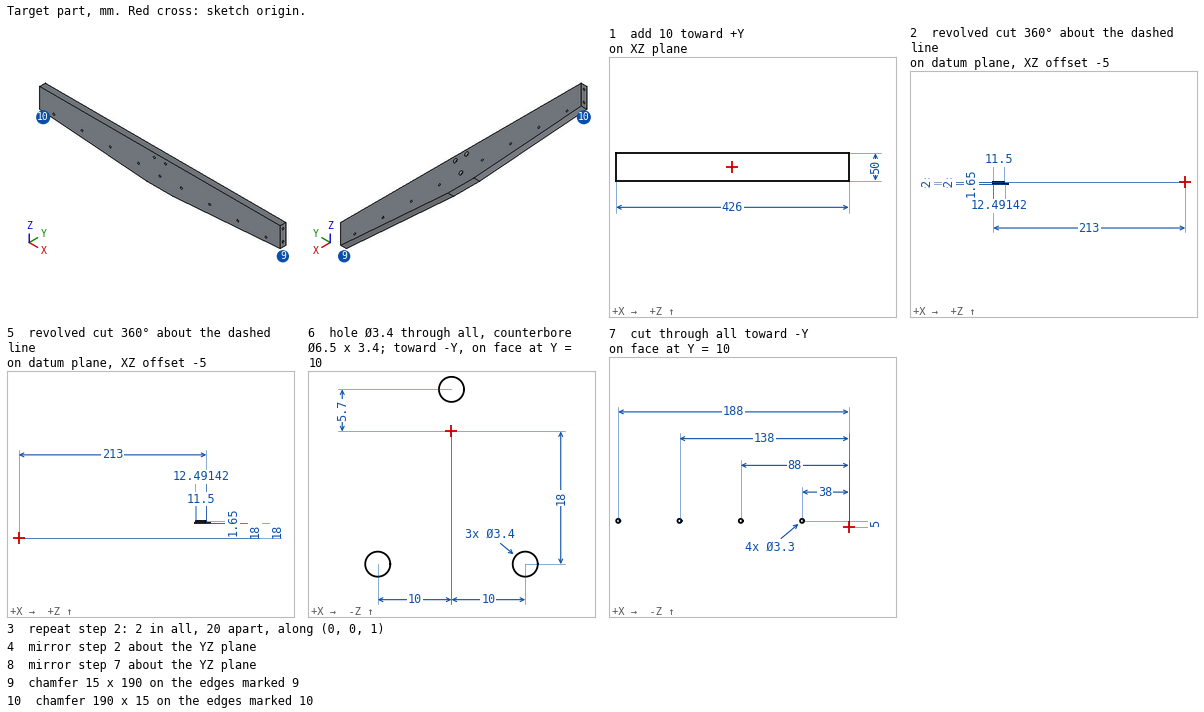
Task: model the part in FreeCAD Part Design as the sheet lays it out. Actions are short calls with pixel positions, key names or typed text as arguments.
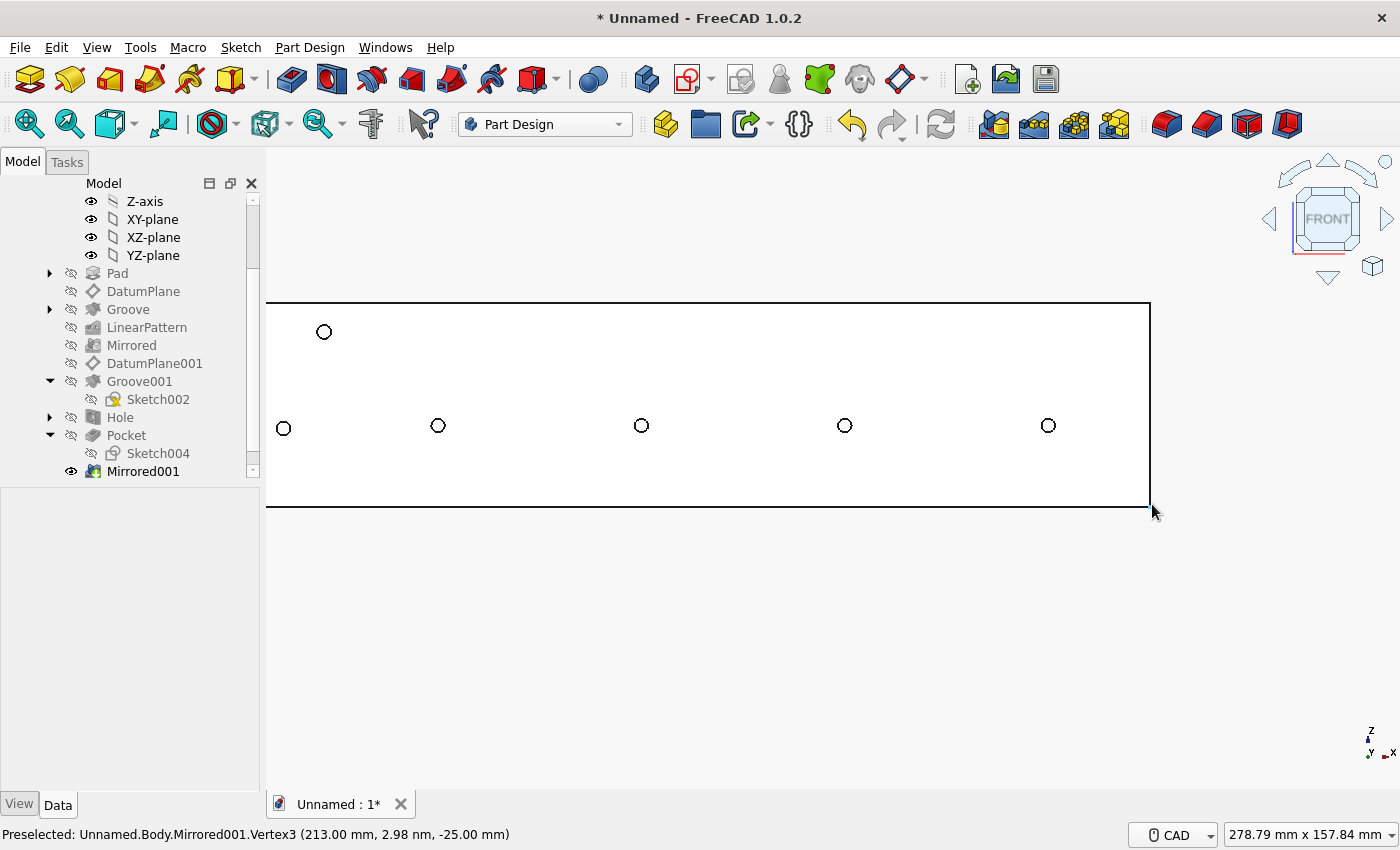
click(30, 124)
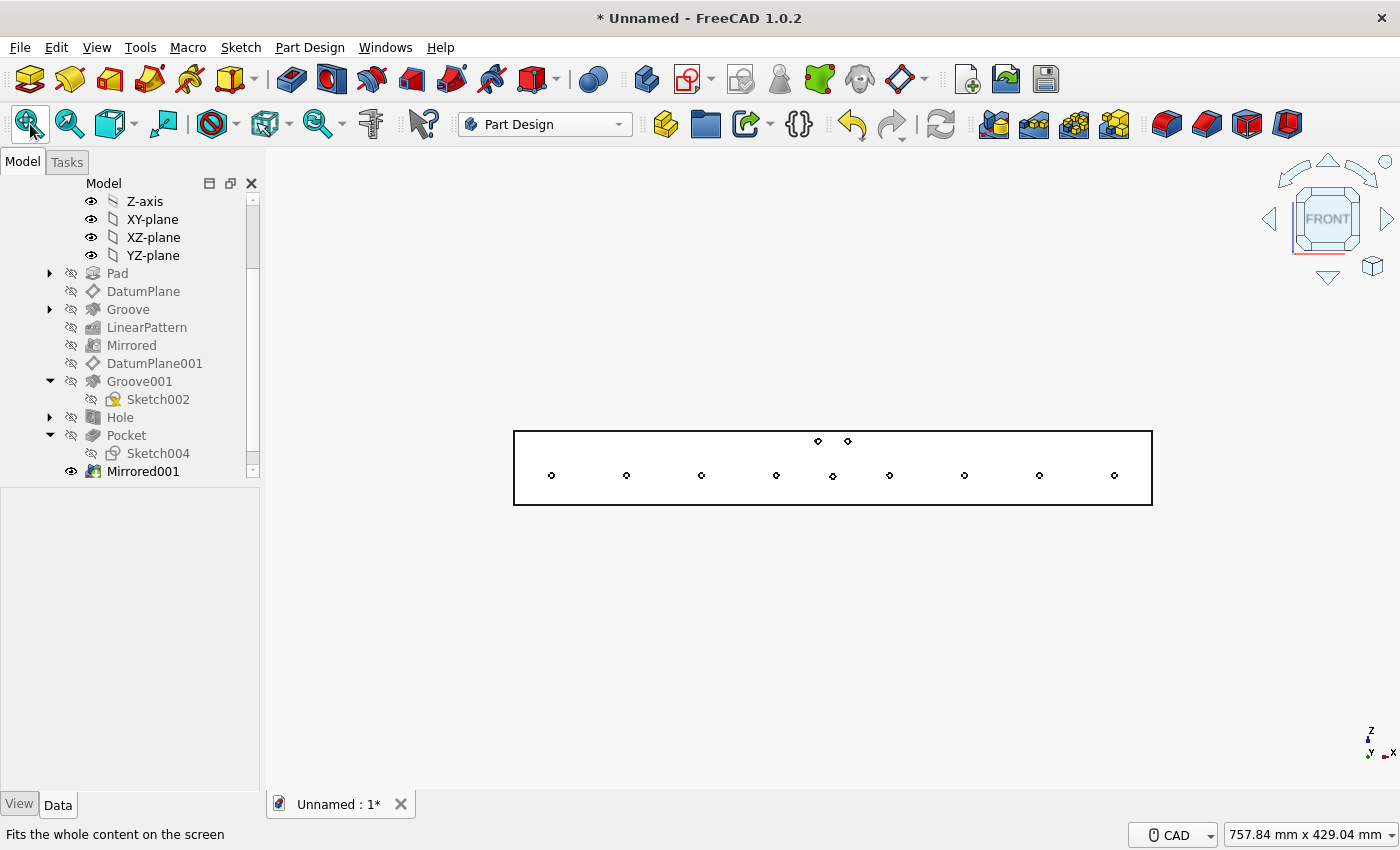
key(3)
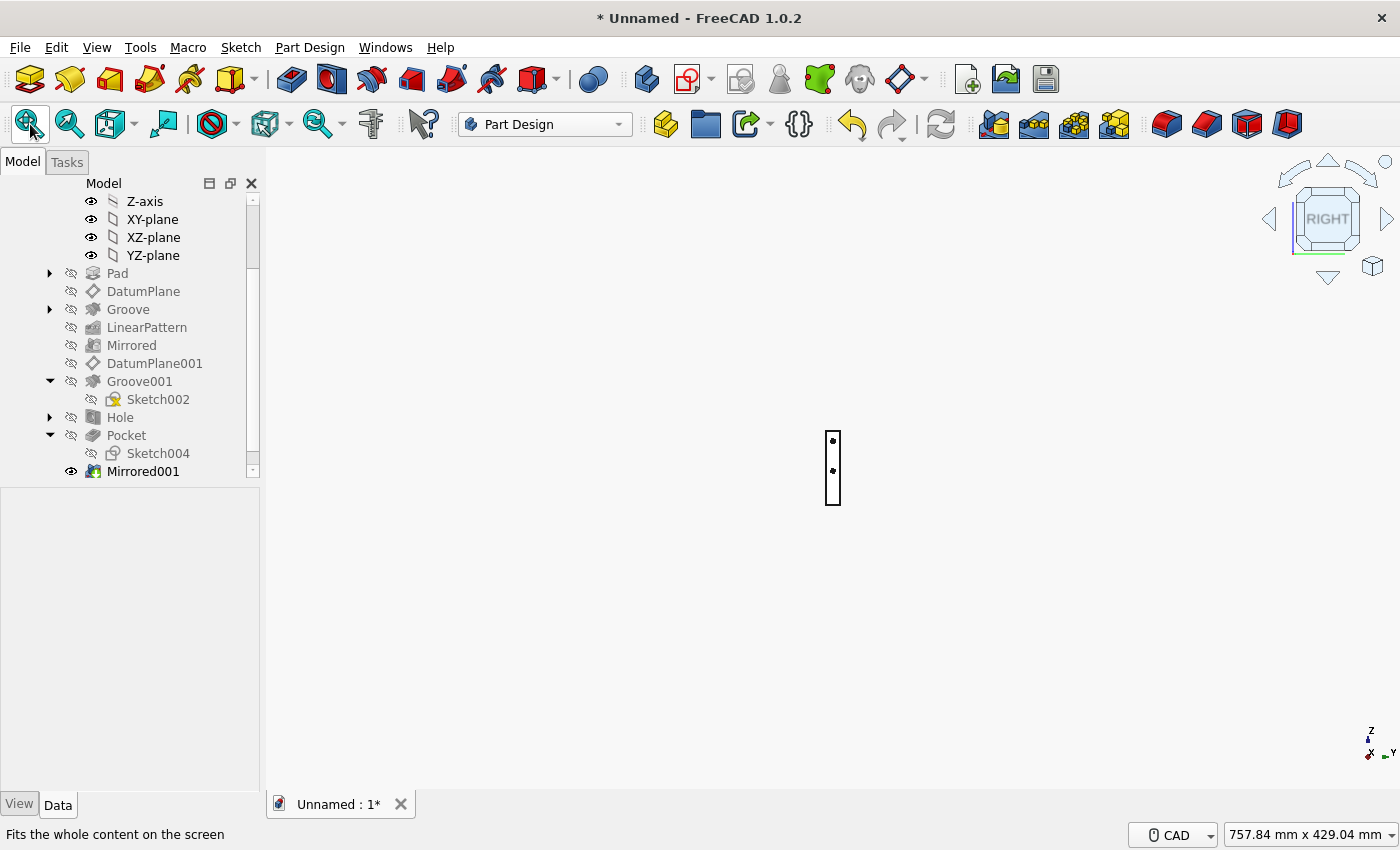
click(30, 124)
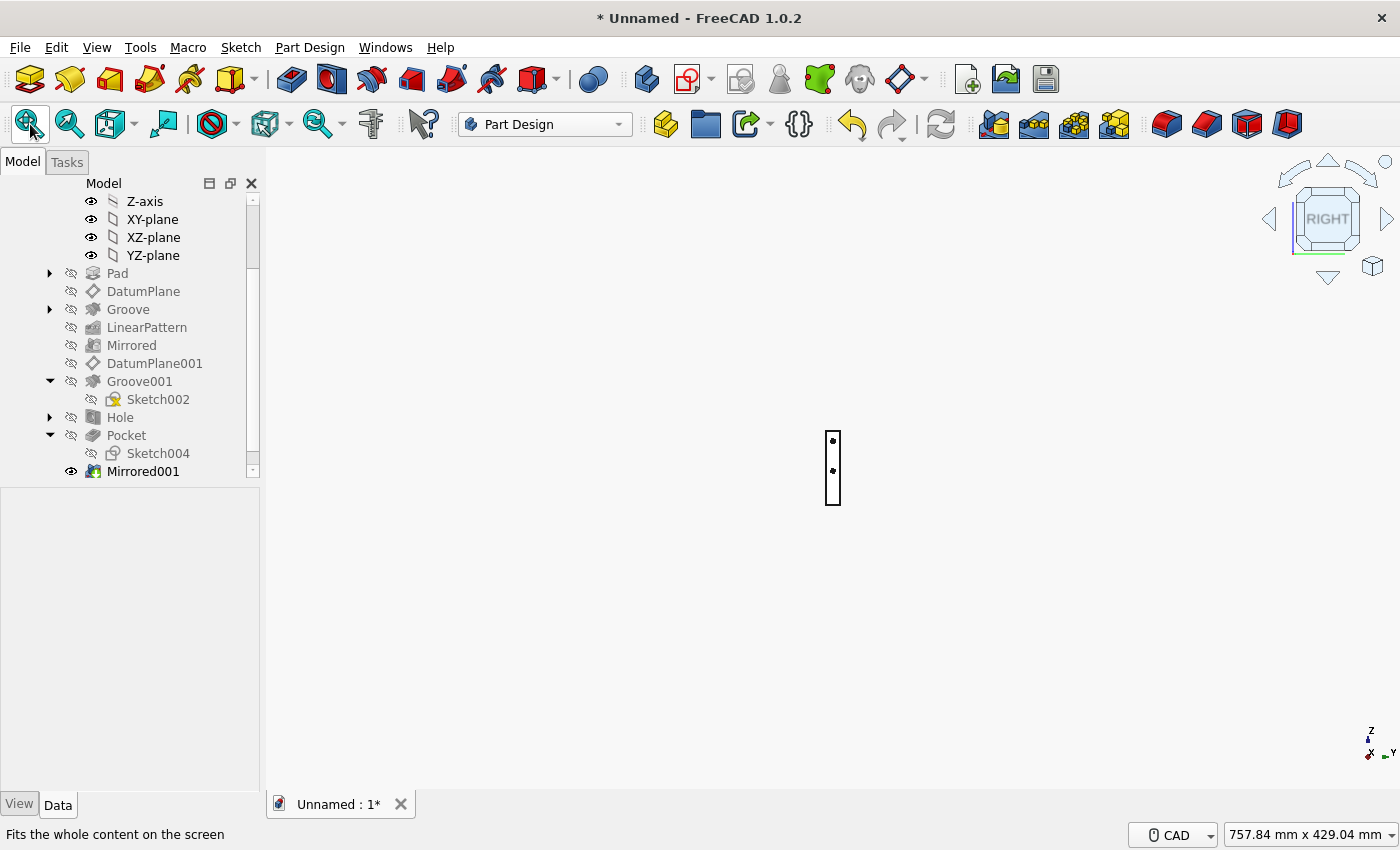
click(833, 504)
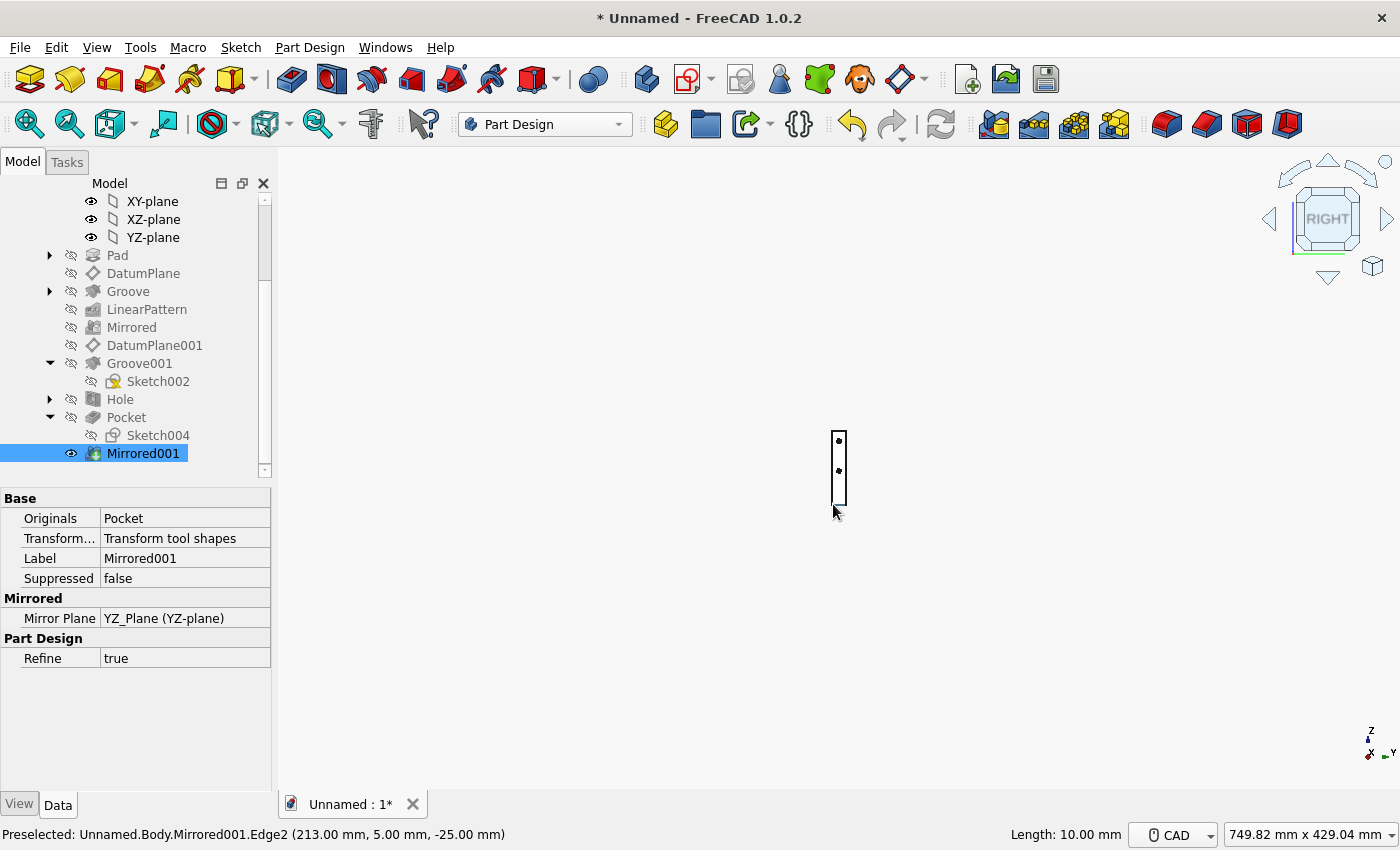
click(1208, 124)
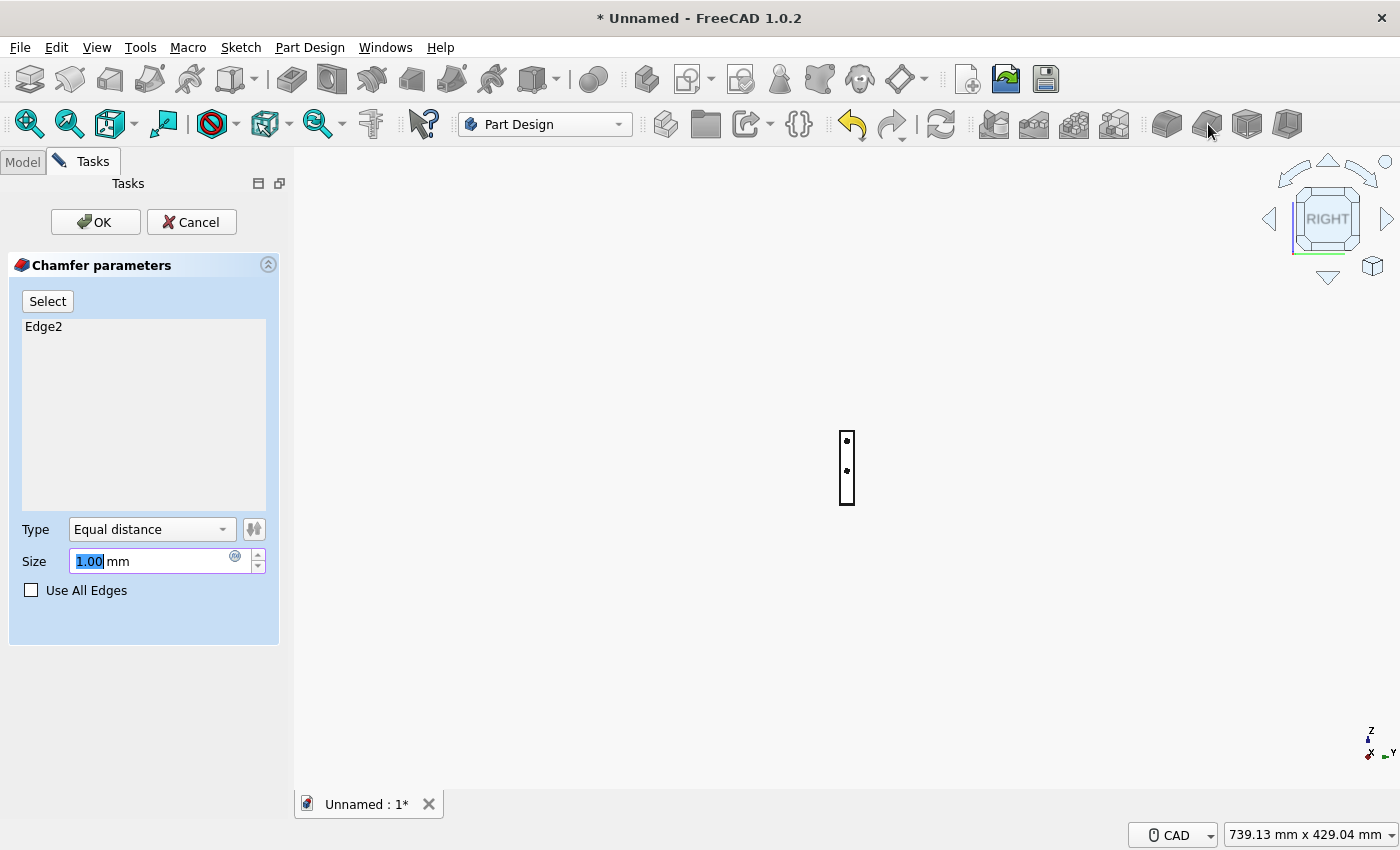
text(15)
key(Tab)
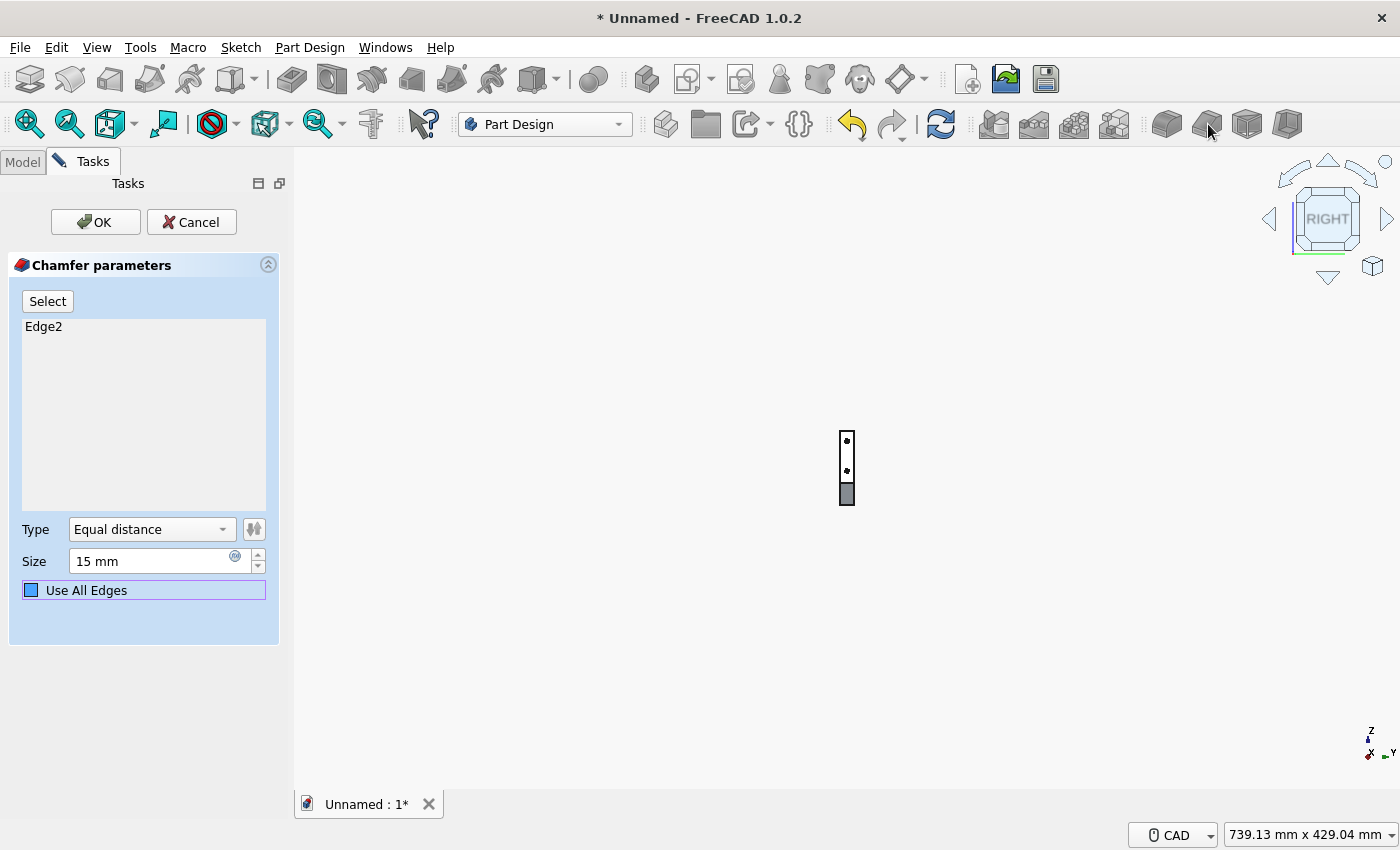
click(153, 530)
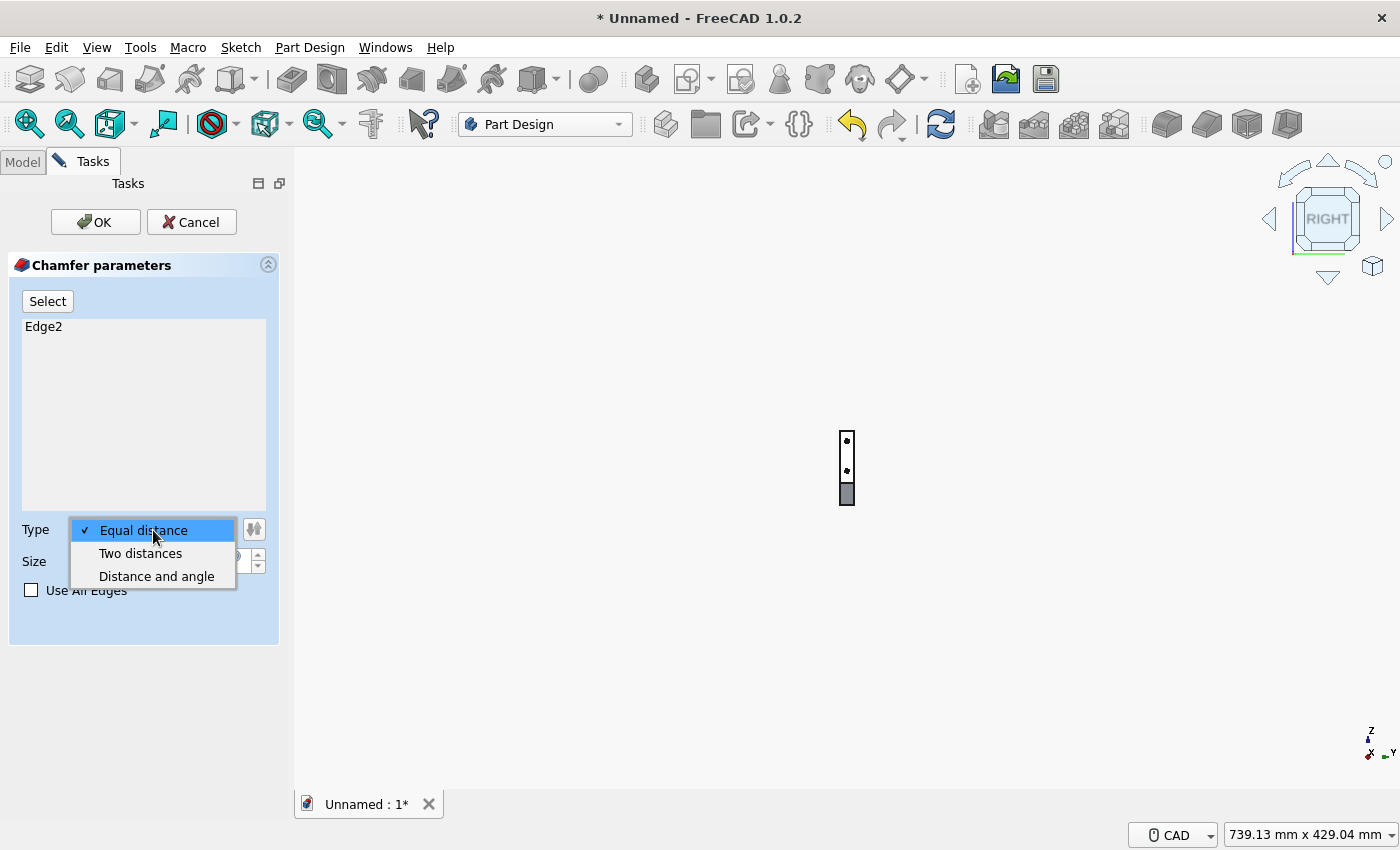
click(152, 554)